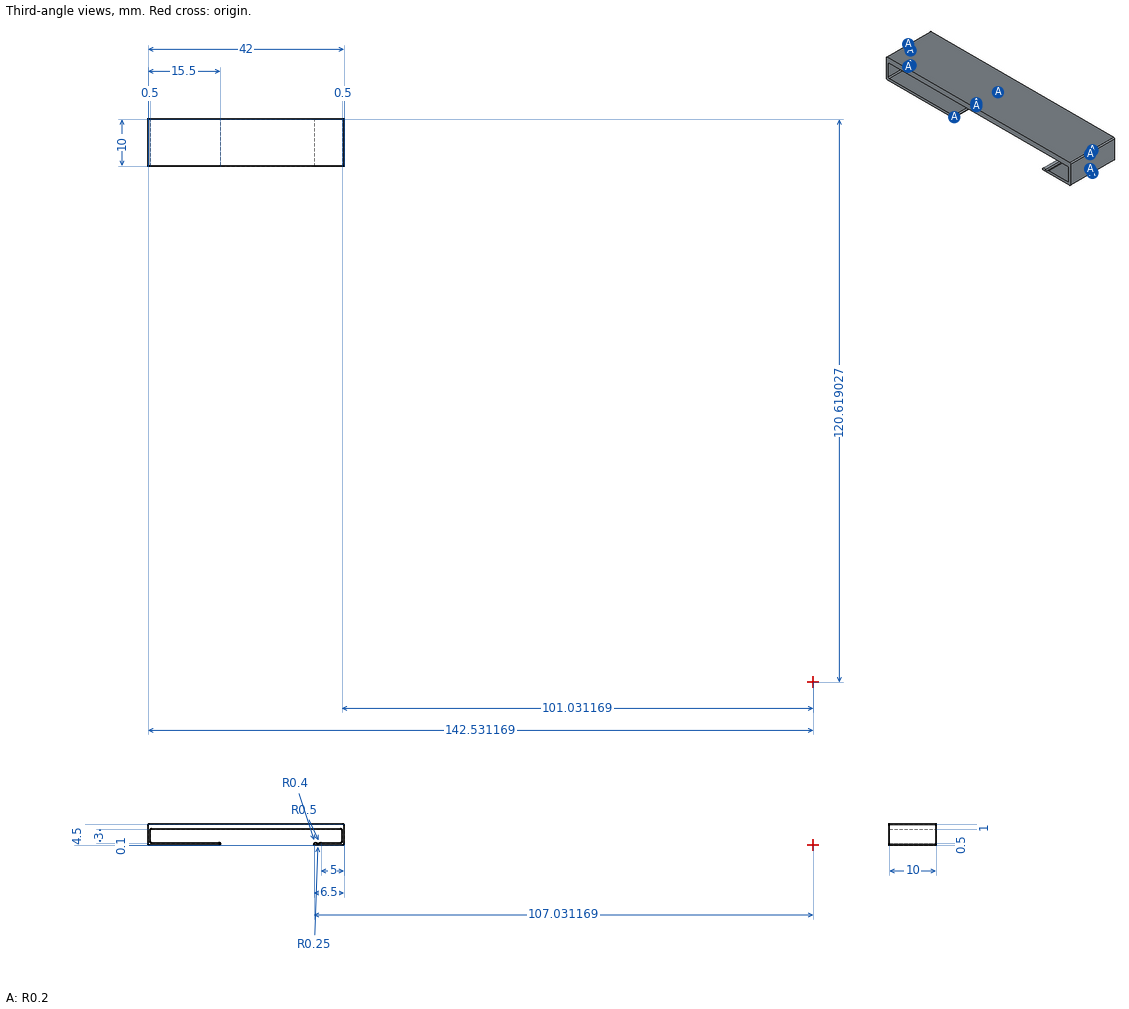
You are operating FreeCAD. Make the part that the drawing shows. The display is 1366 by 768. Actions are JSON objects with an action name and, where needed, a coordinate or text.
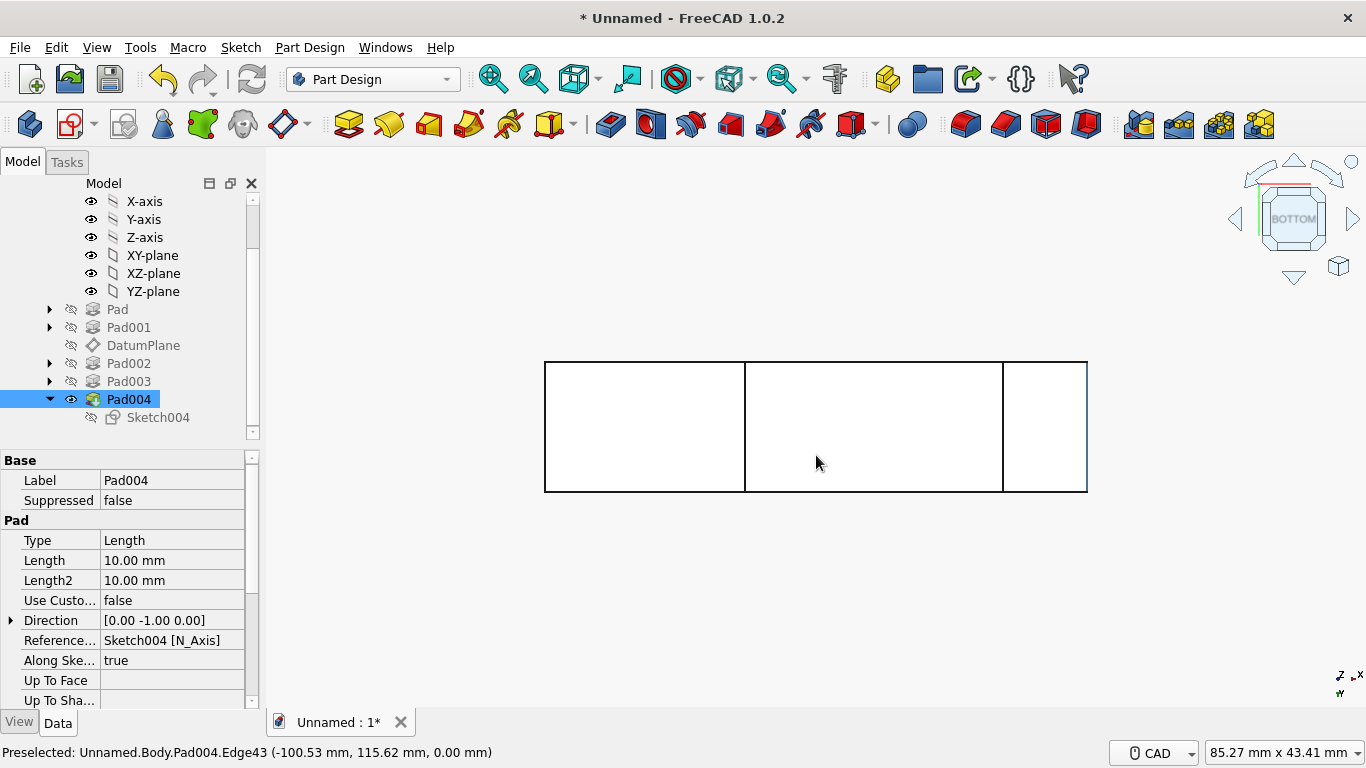
{"action": "left_click", "coordinate": [545, 426], "text": "ctrl"}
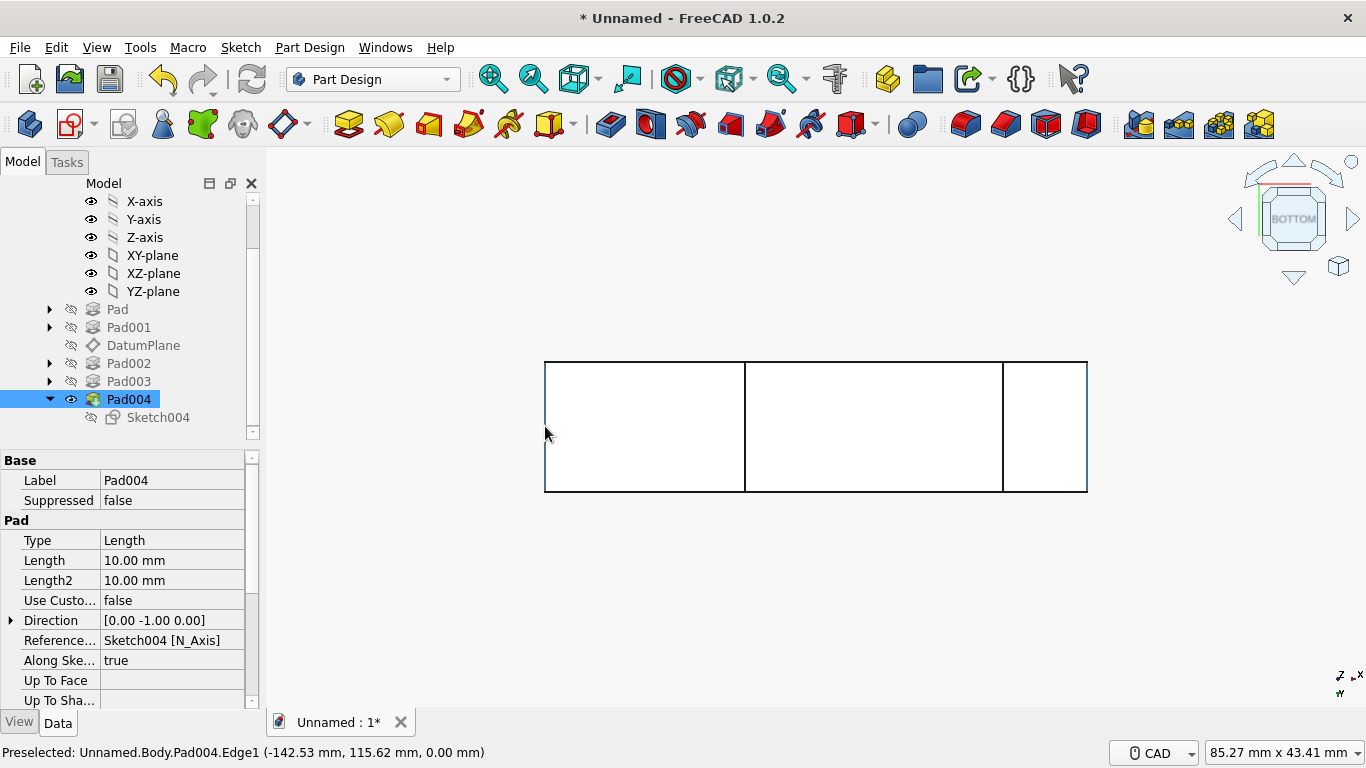
{"action": "key", "text": "4"}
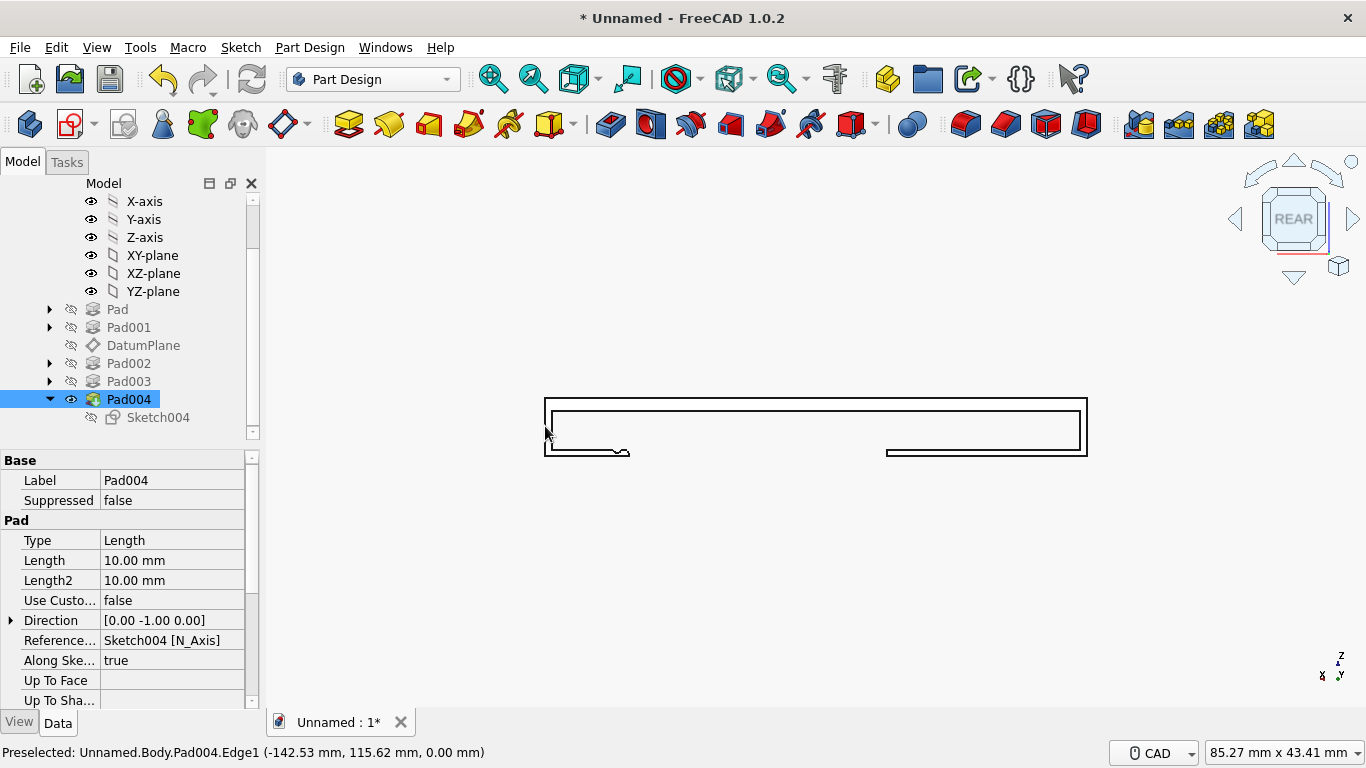
{"action": "key", "text": "6"}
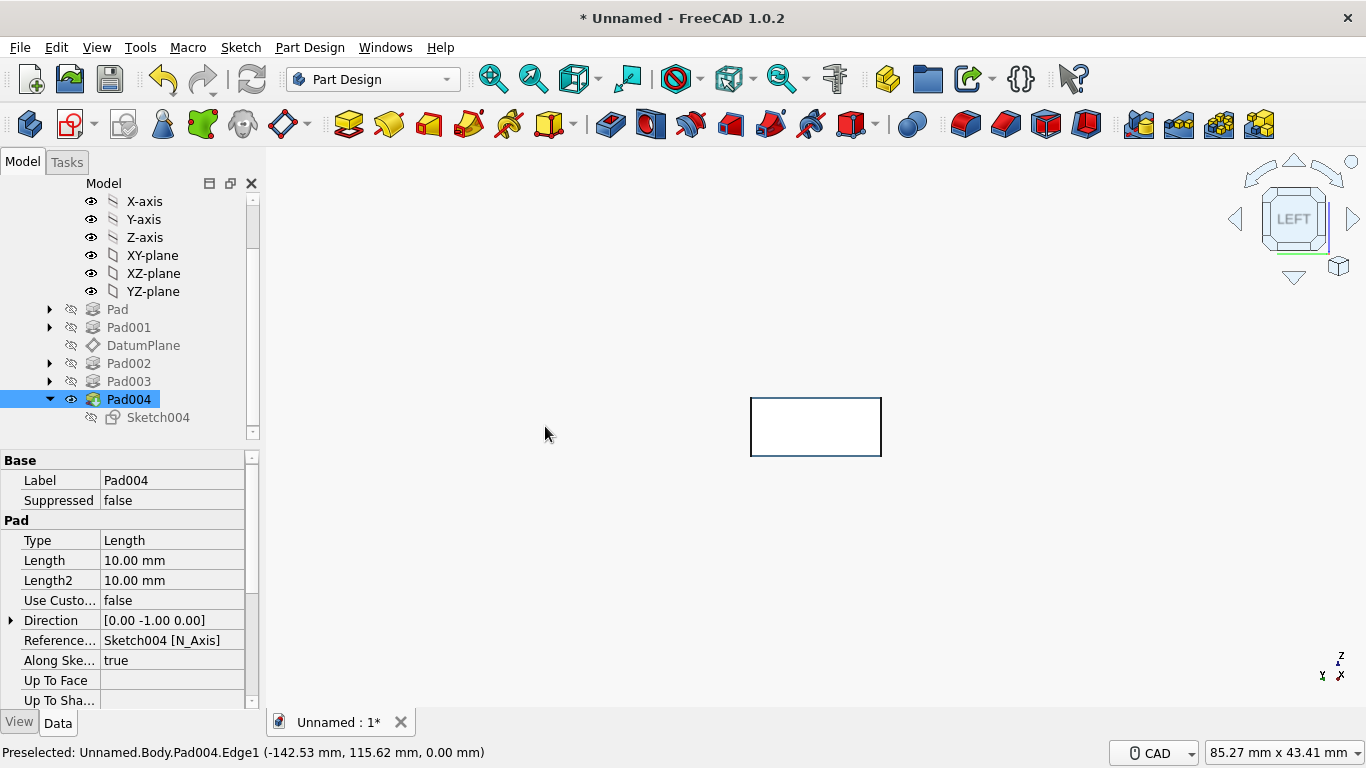
{"action": "left_click", "coordinate": [494, 80]}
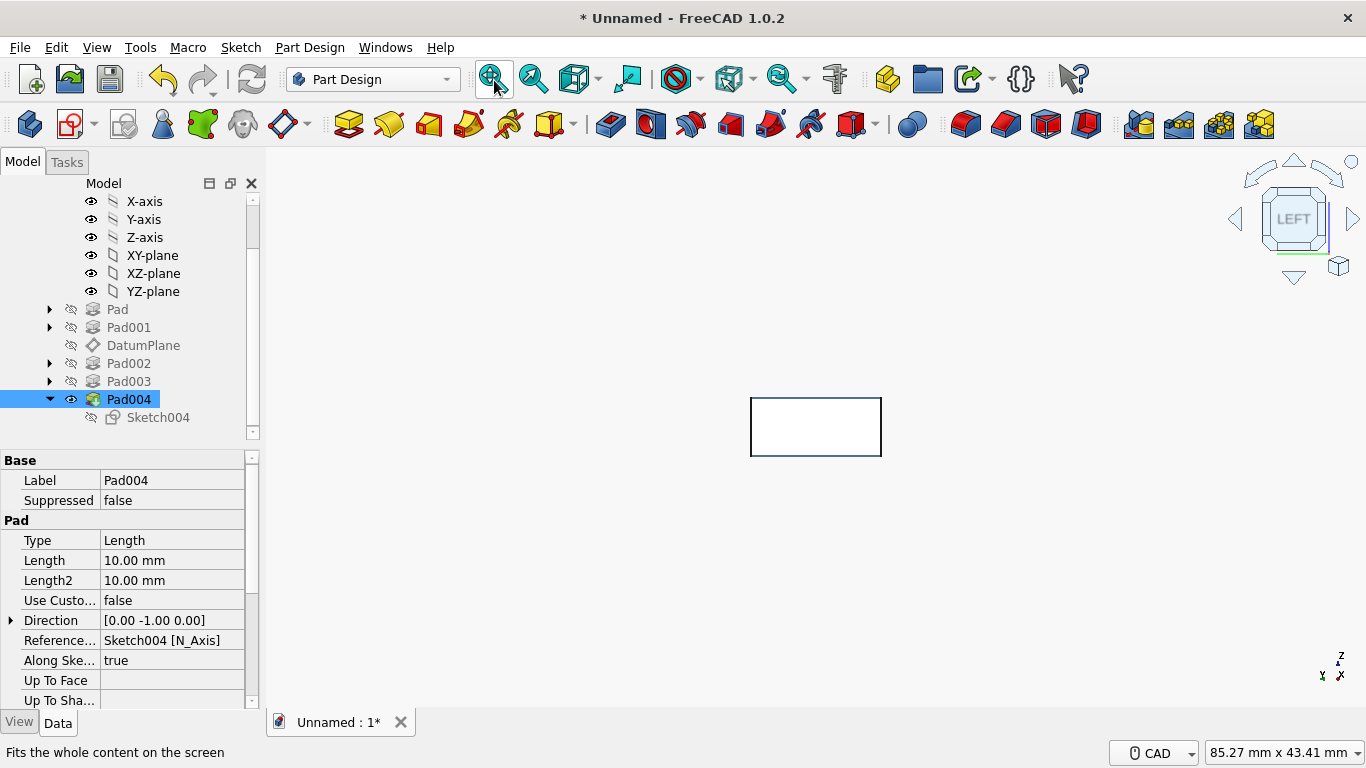
{"action": "key", "text": "v 3"}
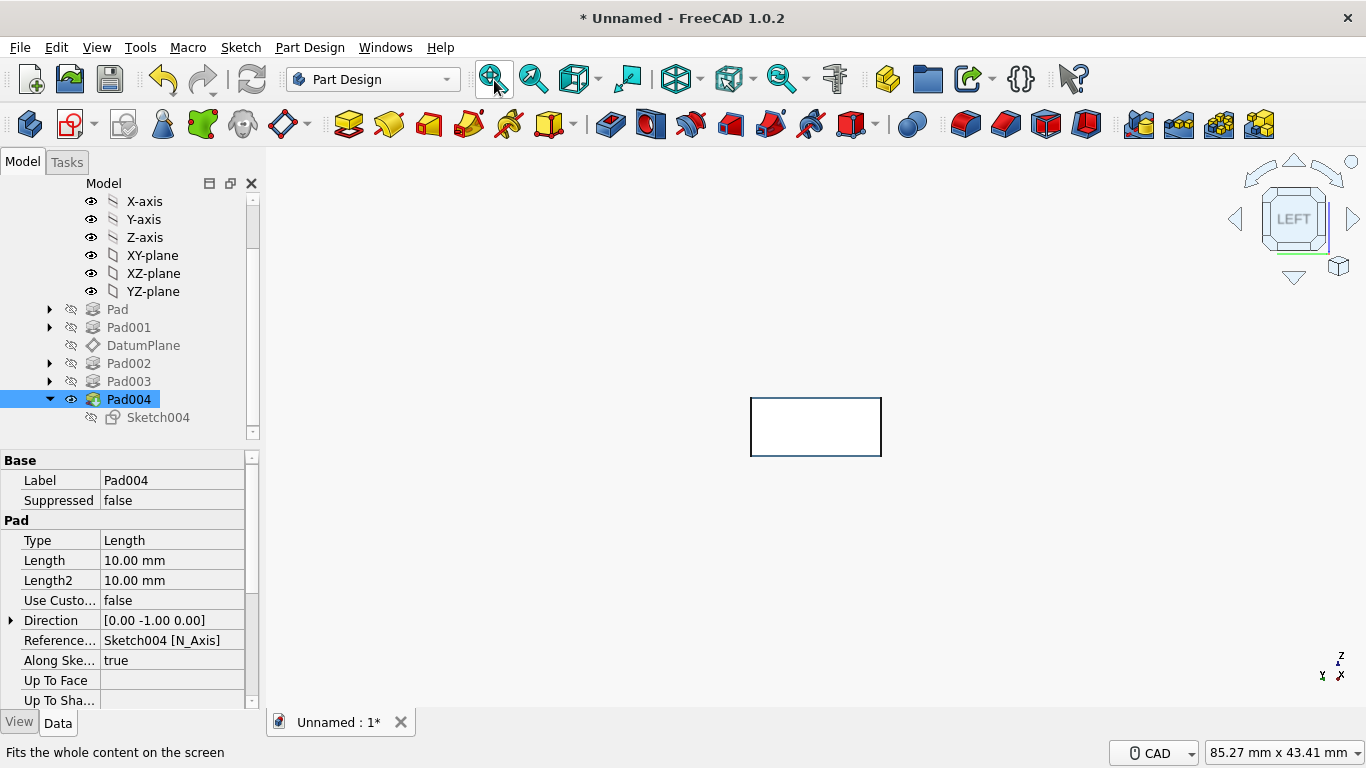
{"action": "key", "text": "0"}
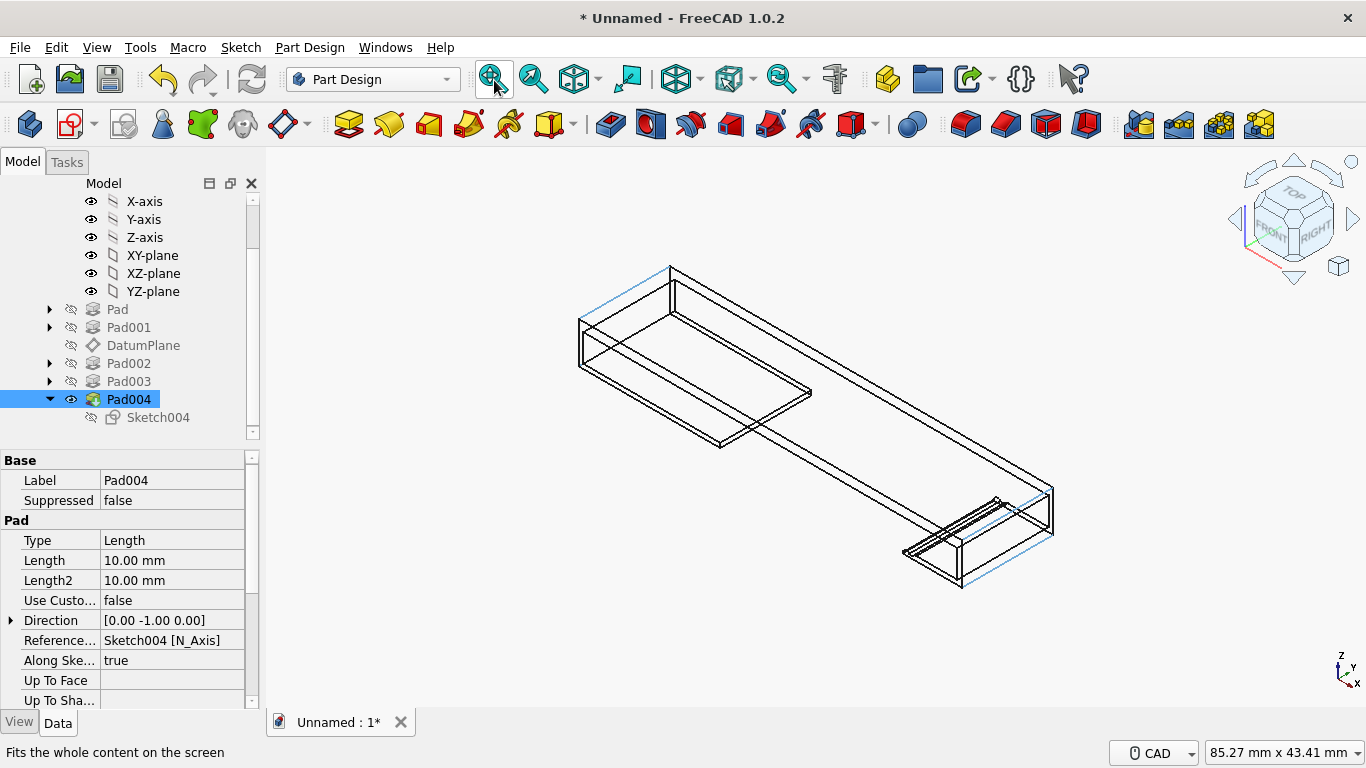
{"action": "left_click", "coordinate": [629, 336], "text": "ctrl"}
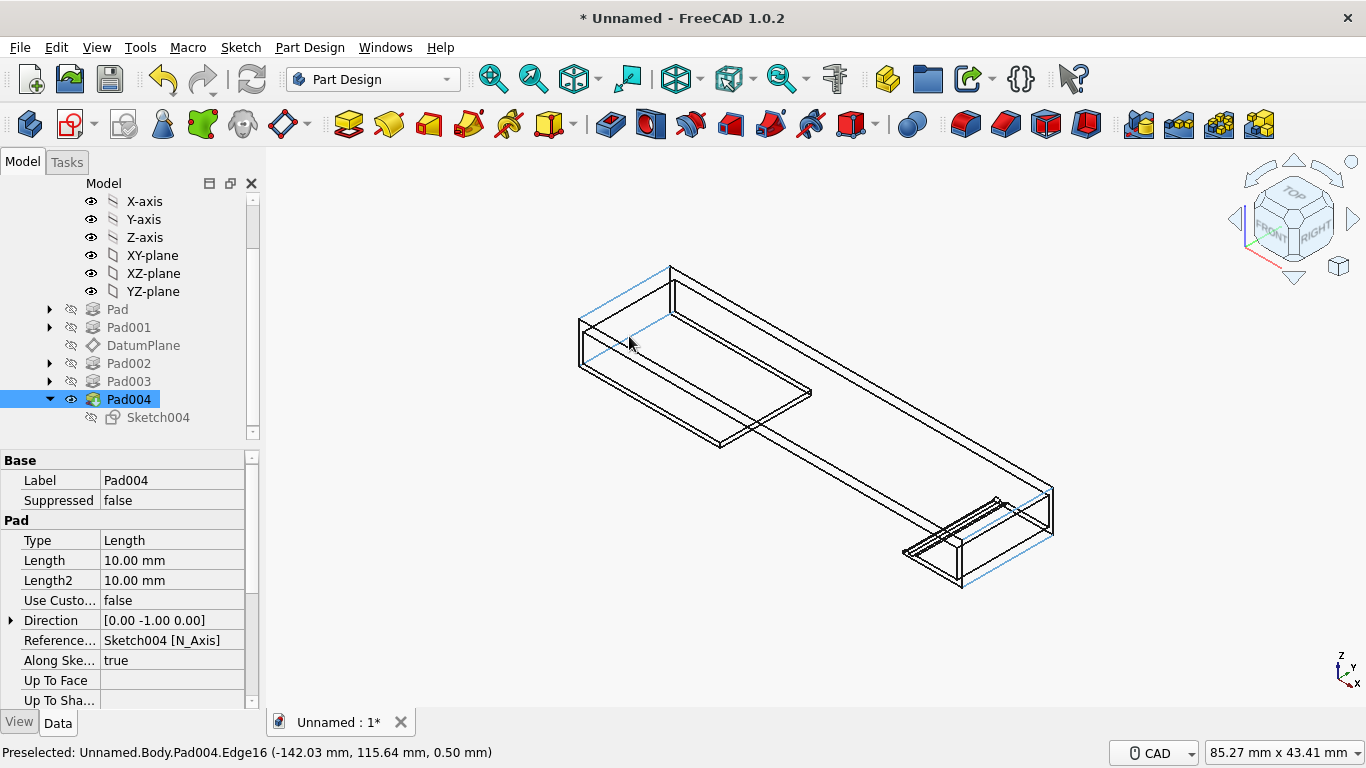
{"action": "left_click", "coordinate": [629, 305], "text": "ctrl"}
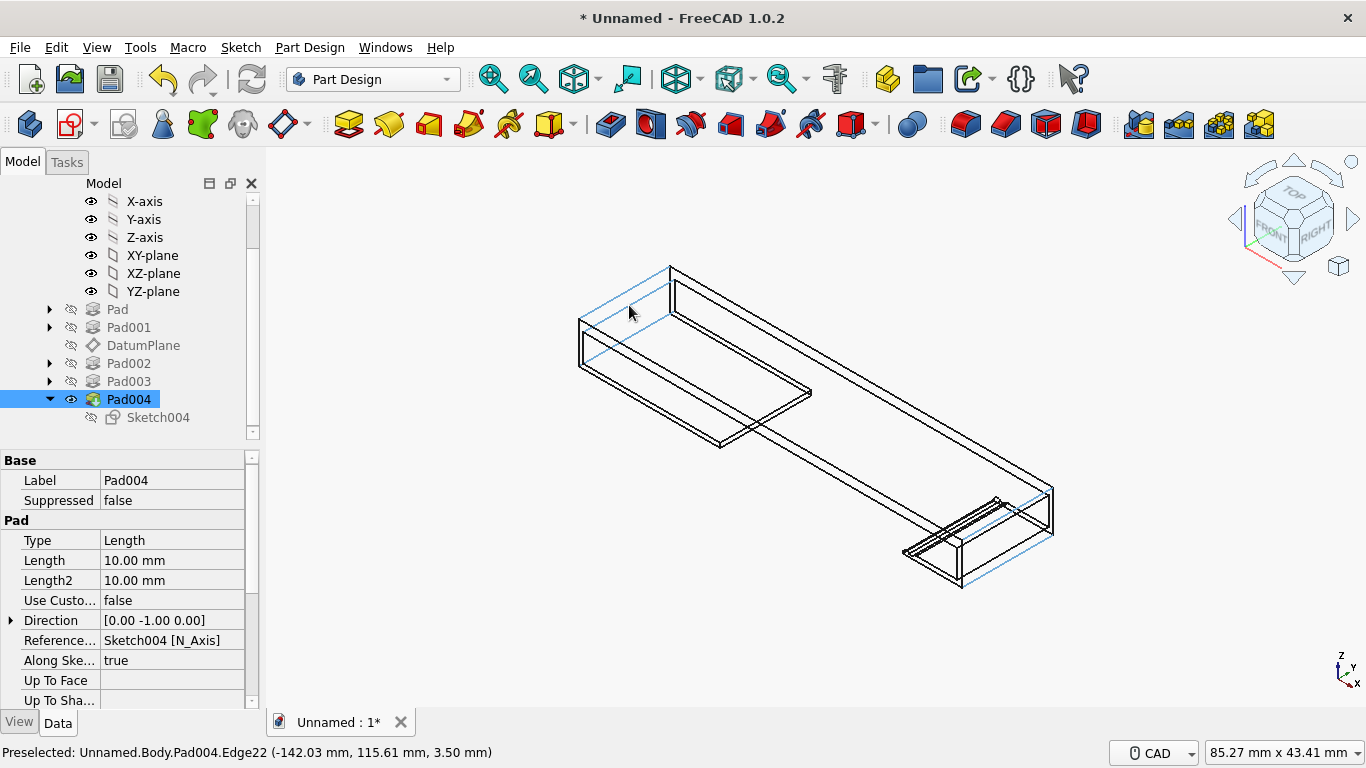
{"action": "left_click", "coordinate": [1003, 552], "text": "ctrl"}